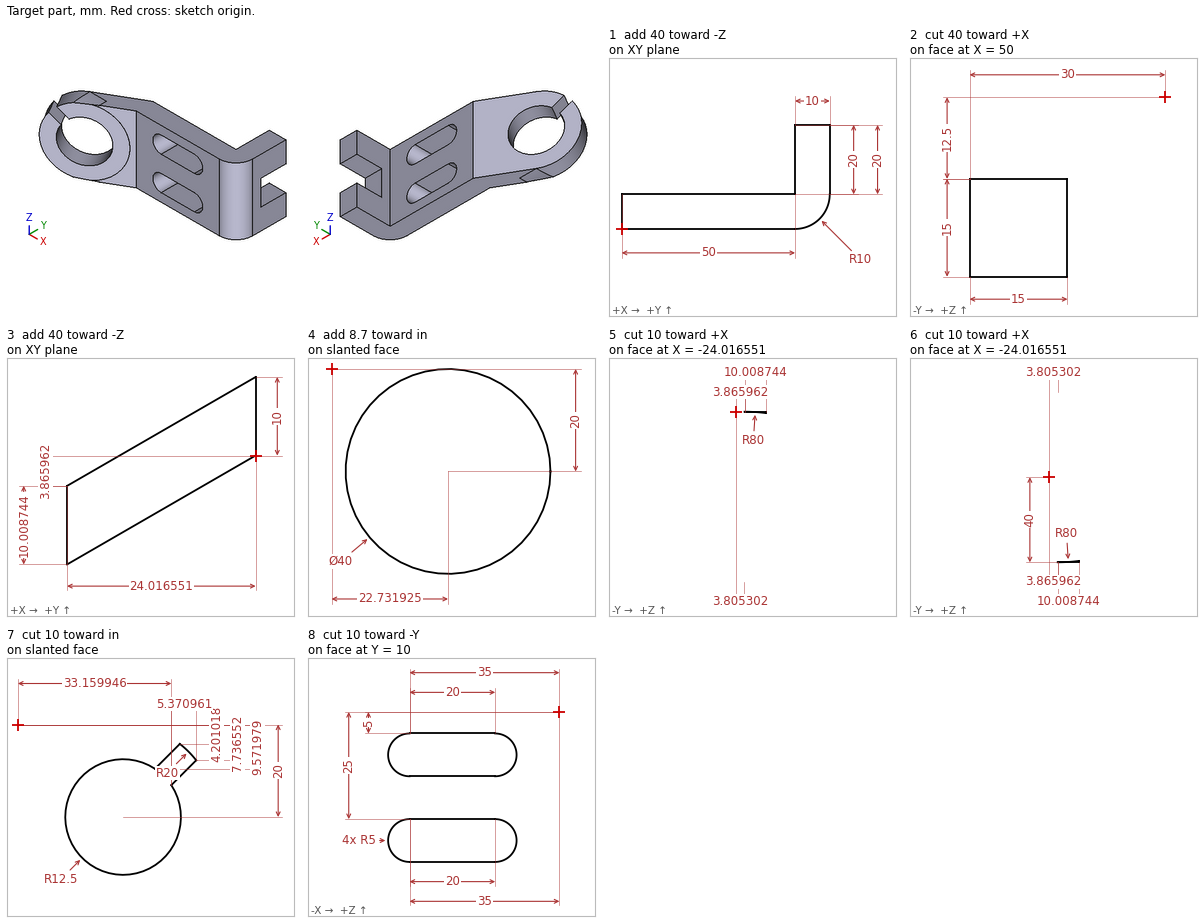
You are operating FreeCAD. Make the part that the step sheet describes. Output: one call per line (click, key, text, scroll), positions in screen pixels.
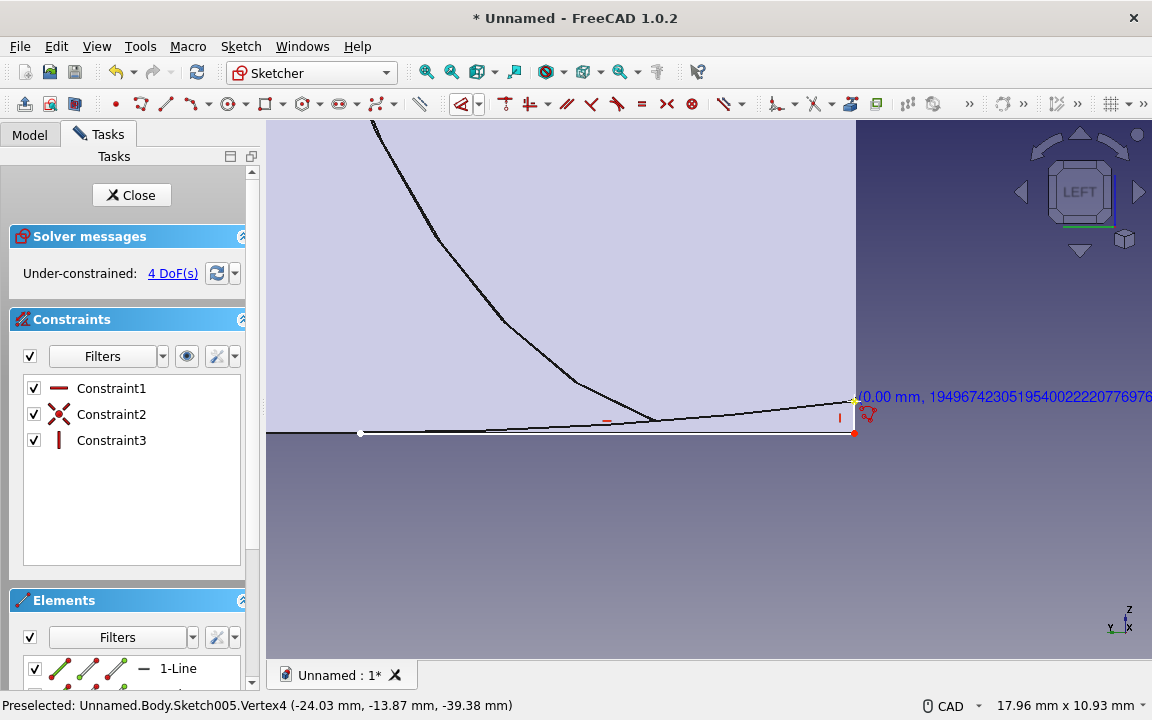
key(g)
key(3)
key(a)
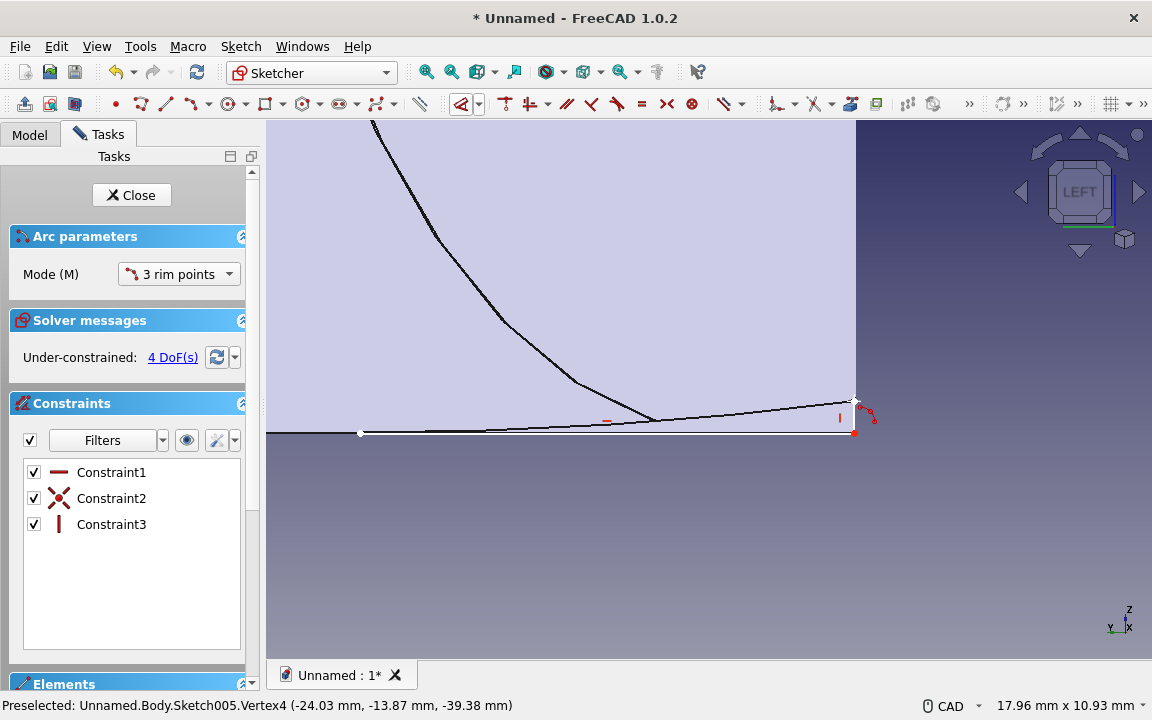
click(854, 402)
click(360, 434)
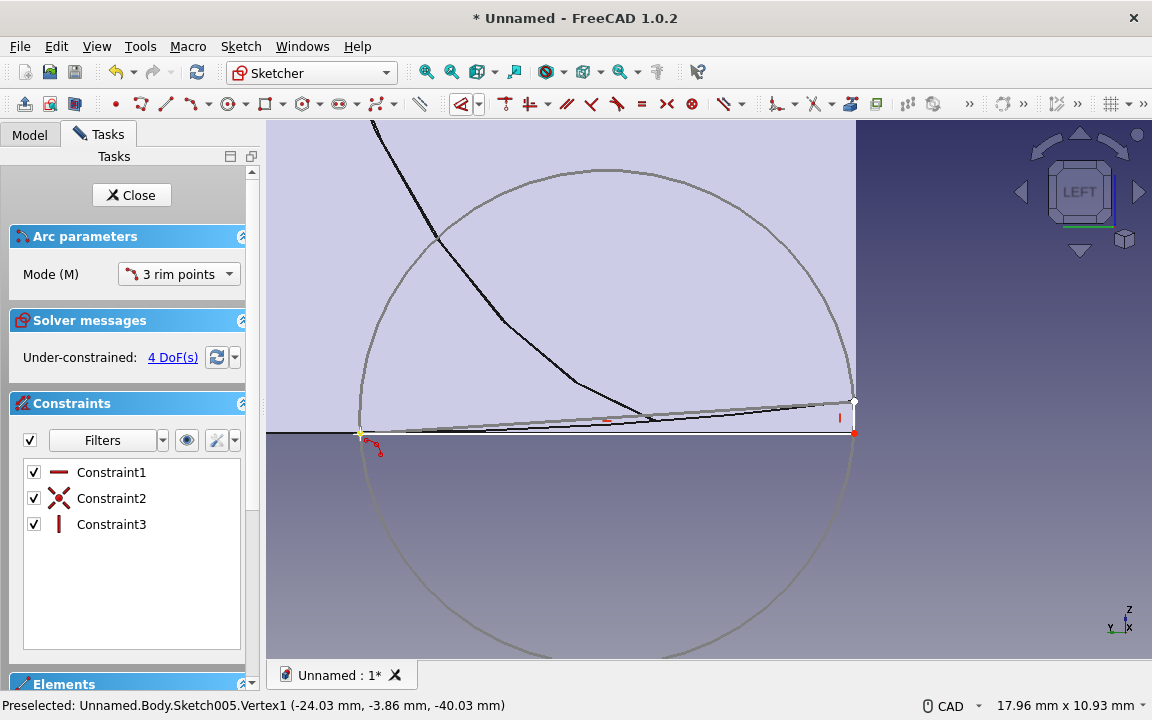
scroll(608, 425, up, 4)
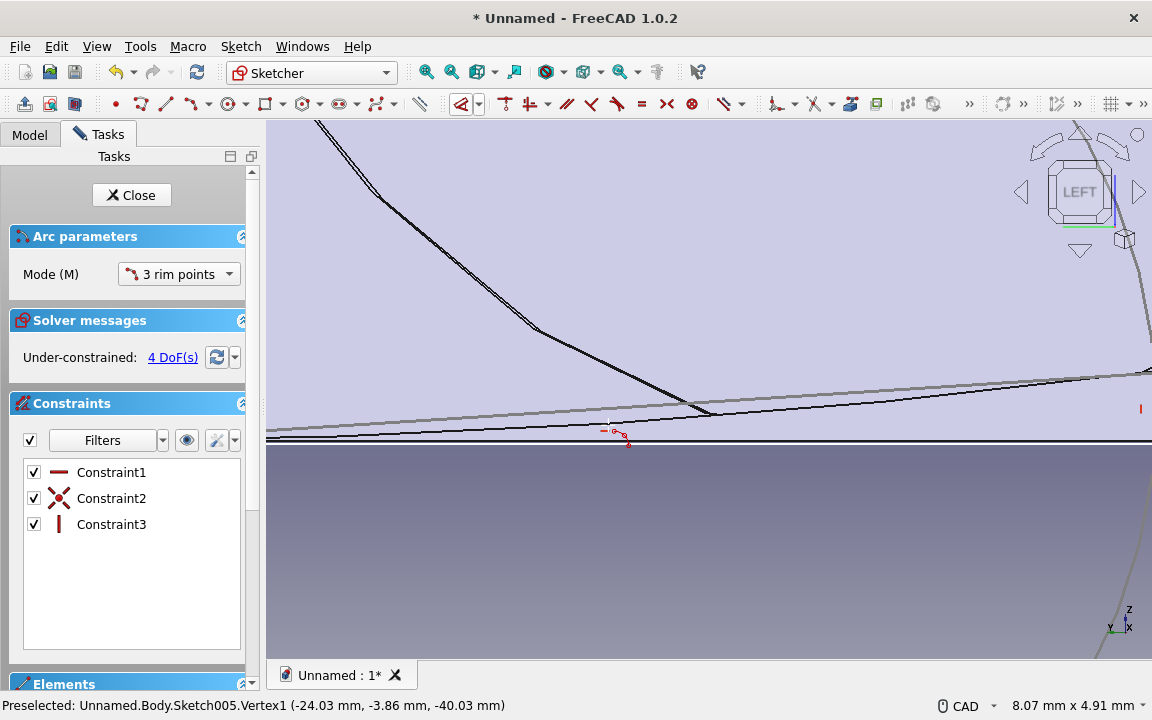
click(607, 423)
key(Escape)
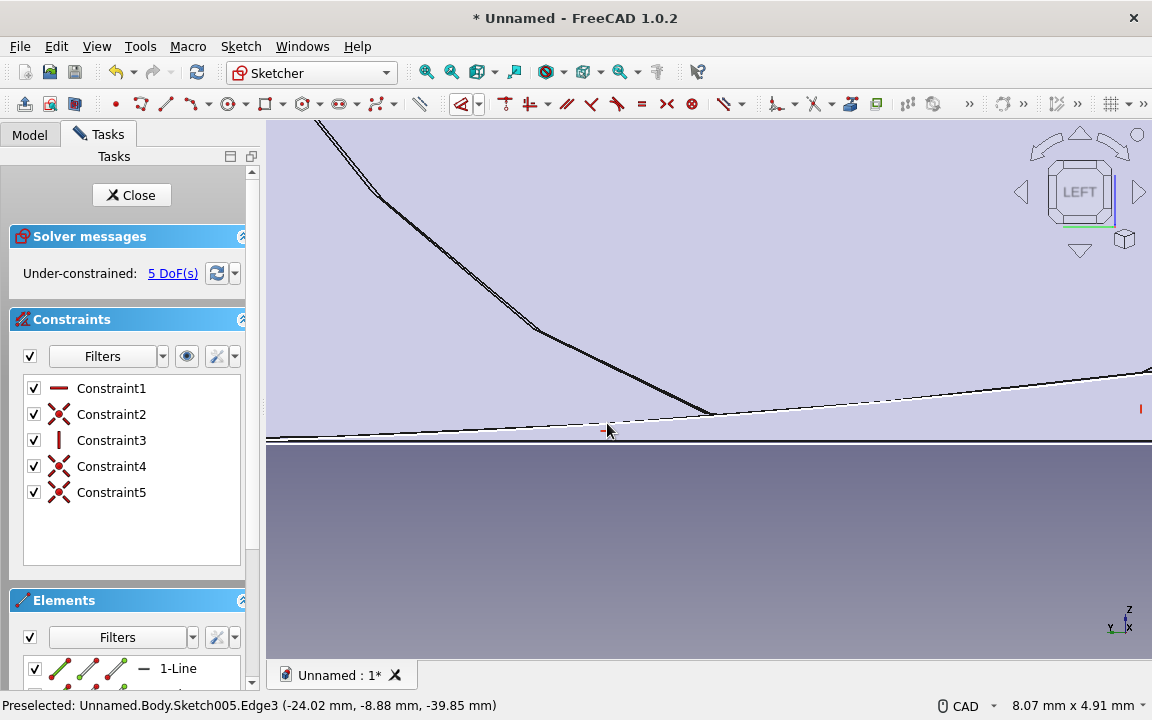
click(826, 407)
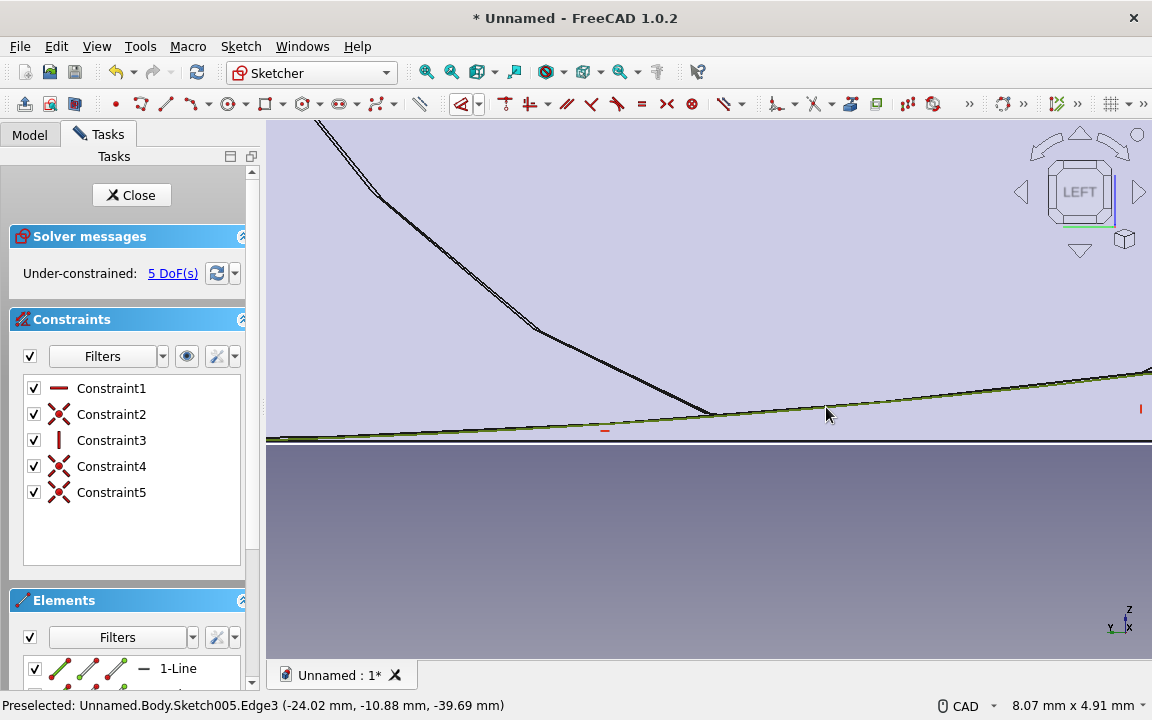
key(k)
key(r)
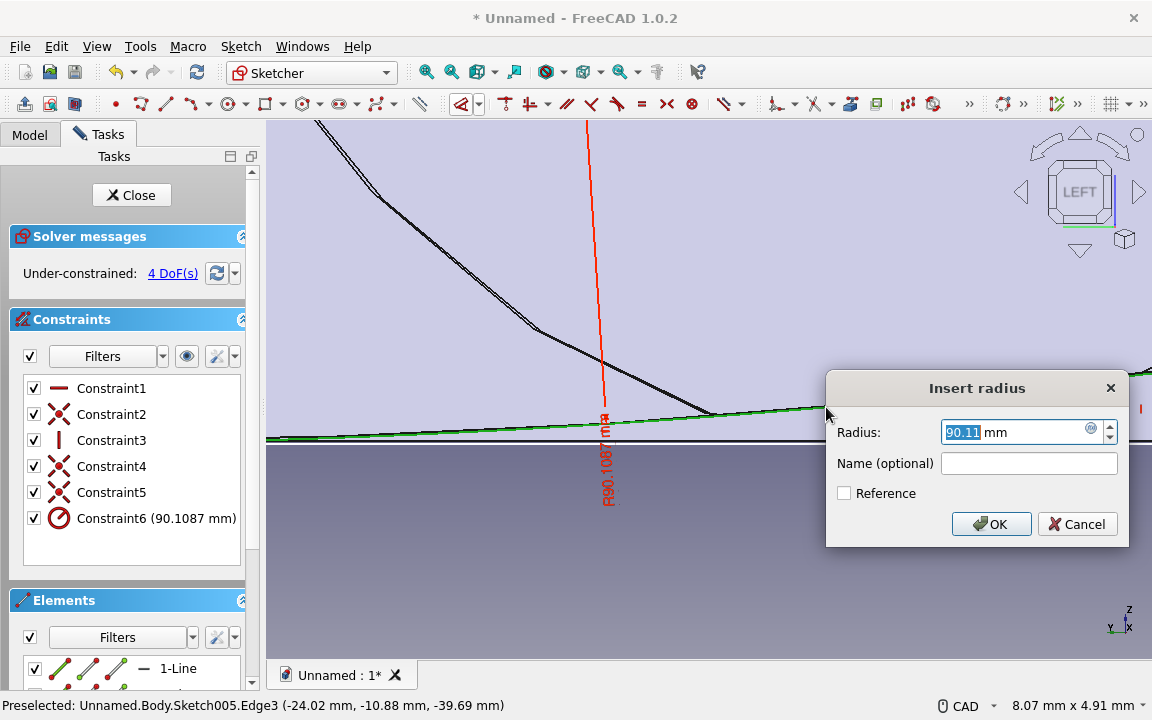
text(80)
key(Return)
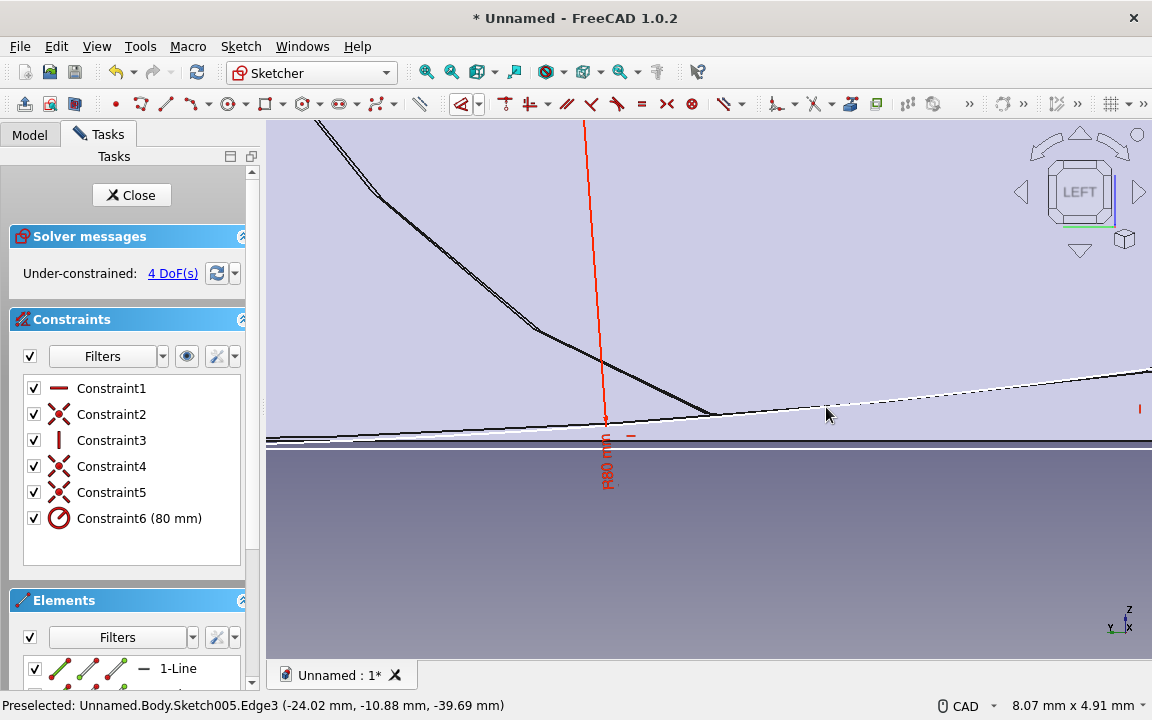
scroll(669, 376, down, 4)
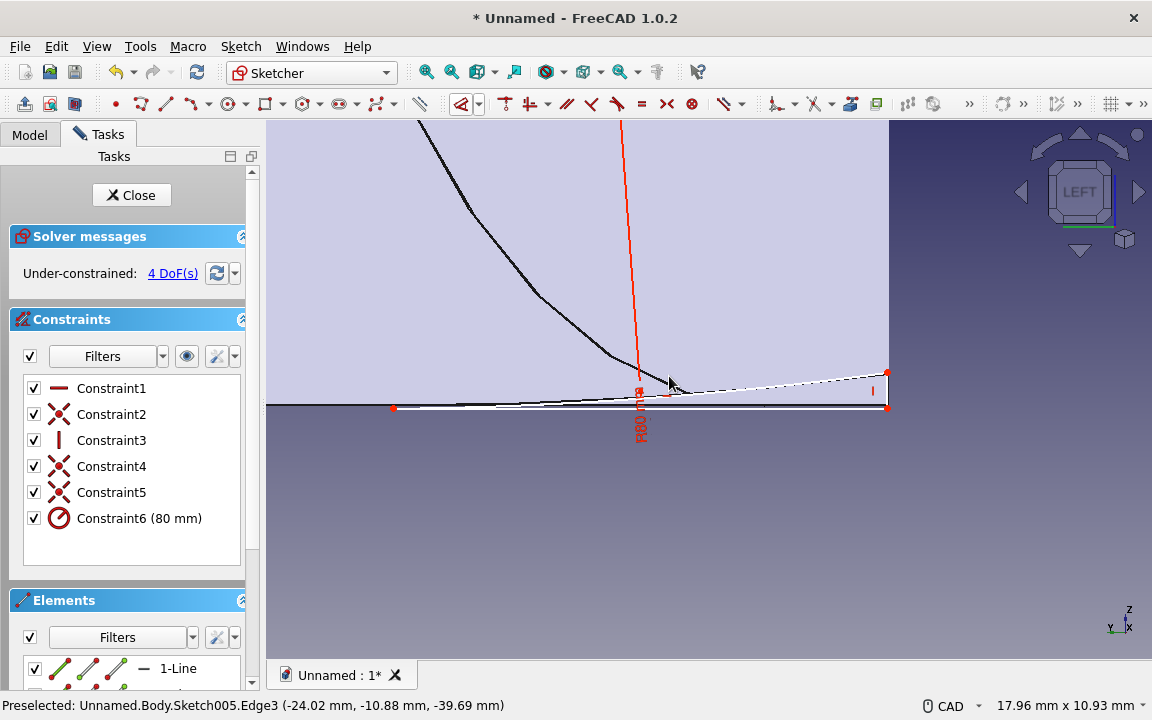
click(394, 409)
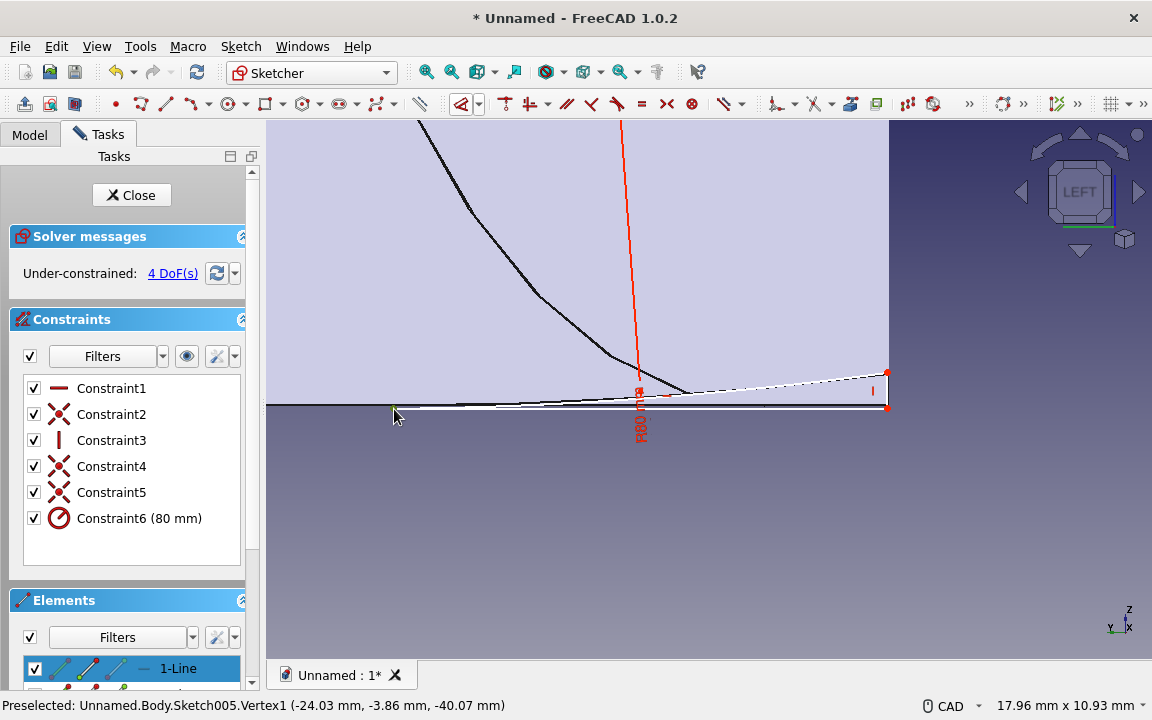
key(i)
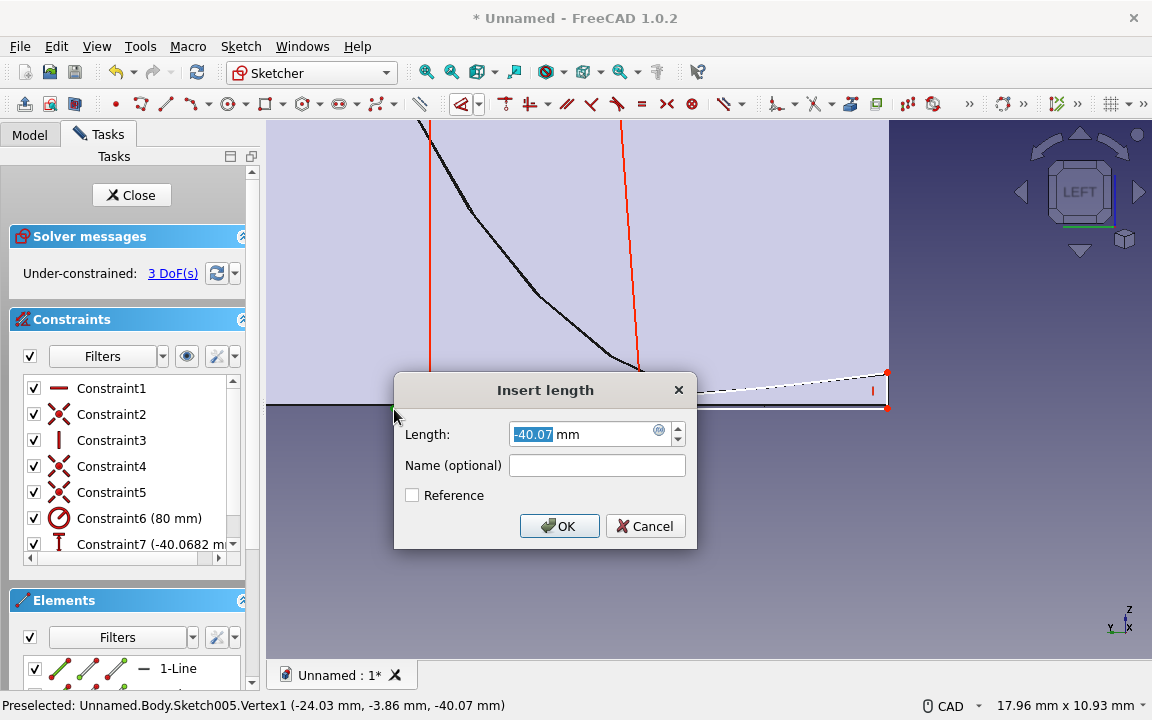
text(-40)
key(Return)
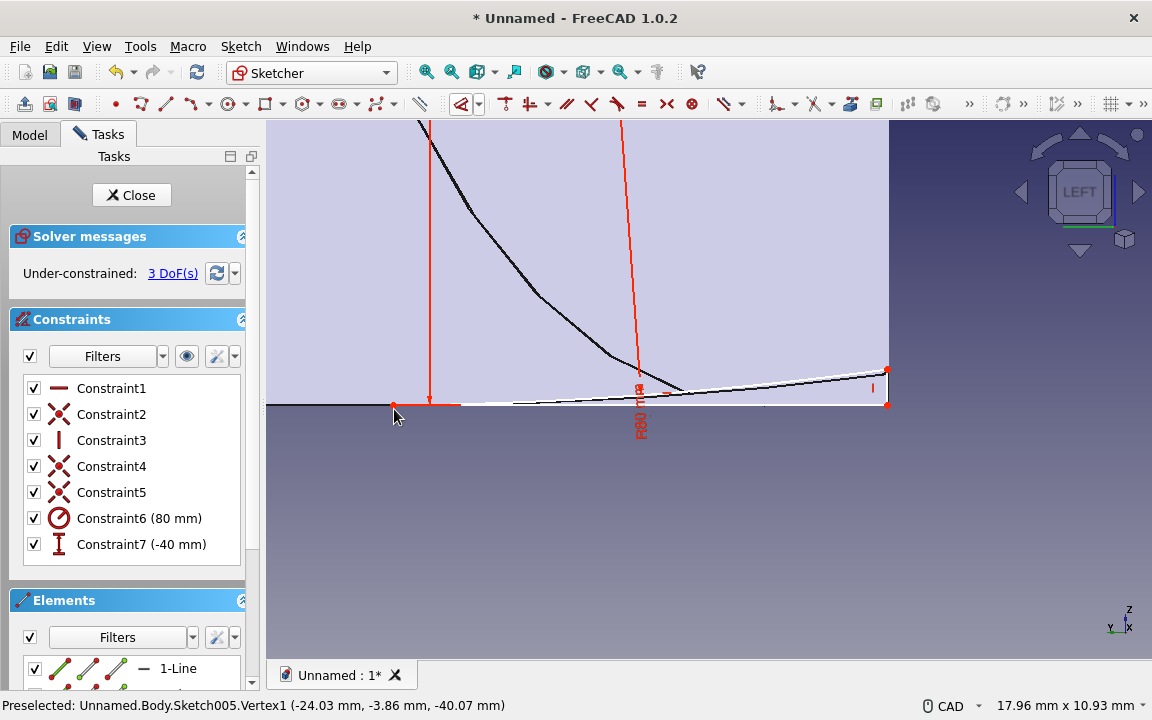
click(739, 405)